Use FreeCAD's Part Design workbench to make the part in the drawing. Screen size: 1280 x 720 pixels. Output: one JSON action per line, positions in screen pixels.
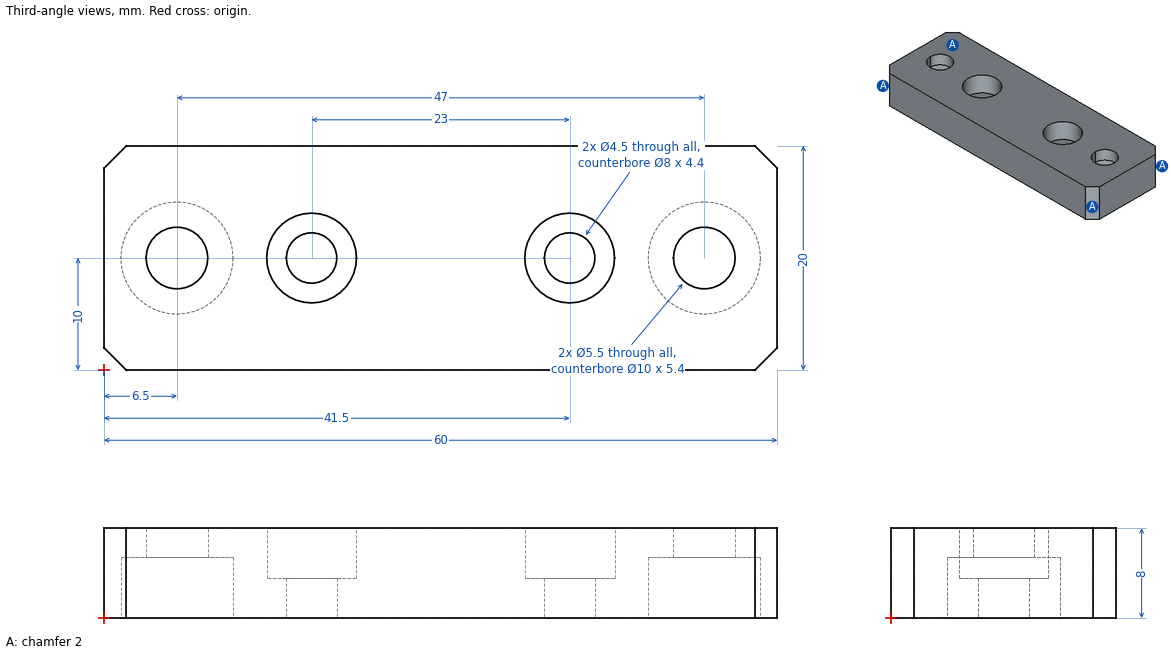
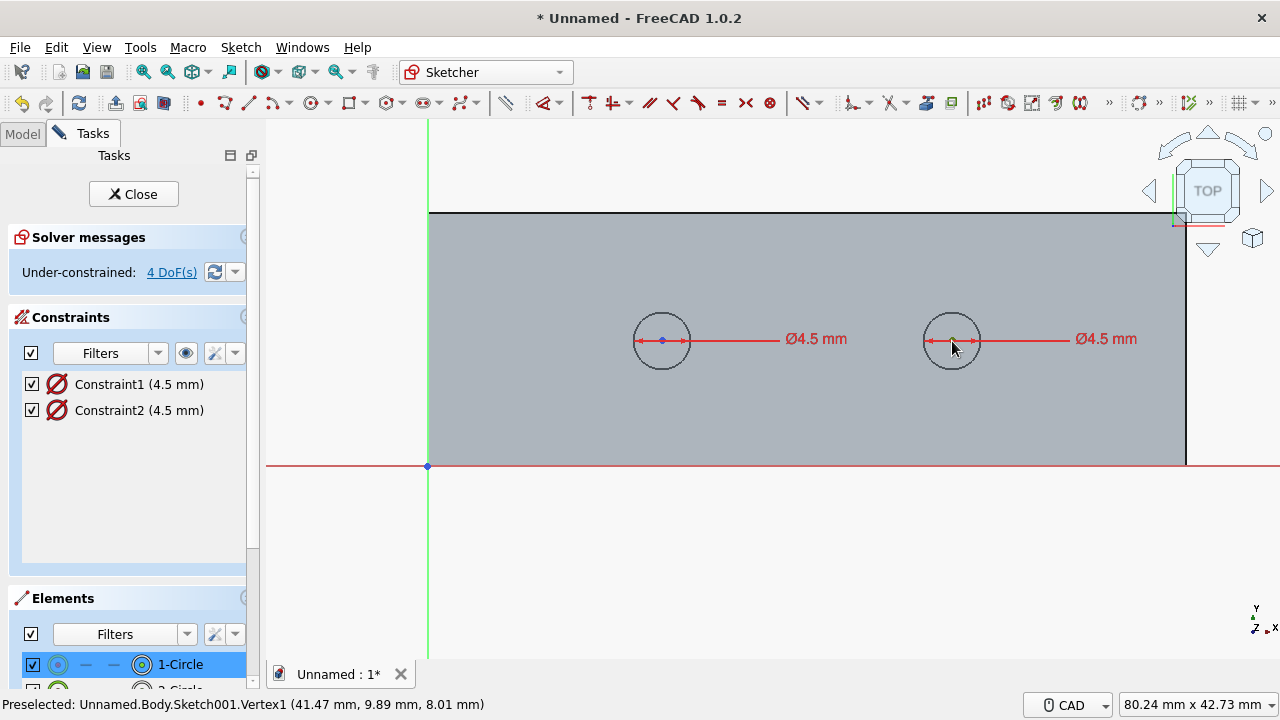
{"action": "left_click", "coordinate": [662, 341]}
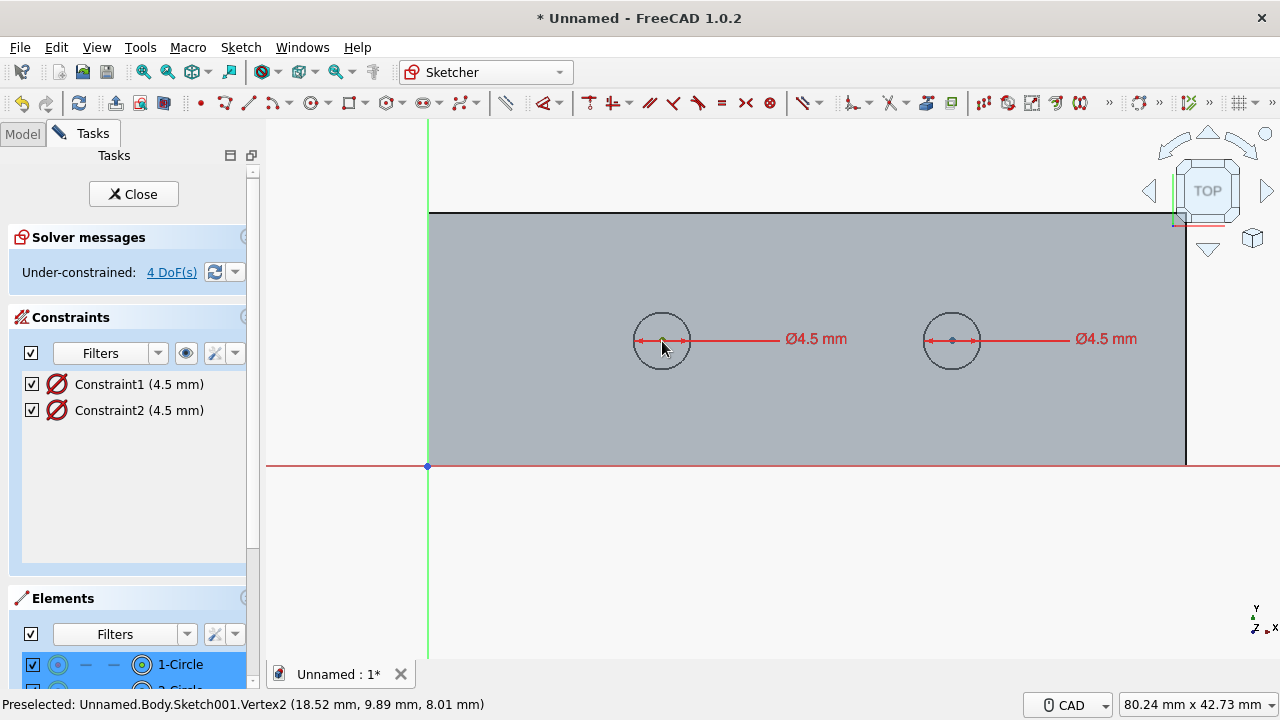
{"action": "left_click", "coordinate": [632, 104]}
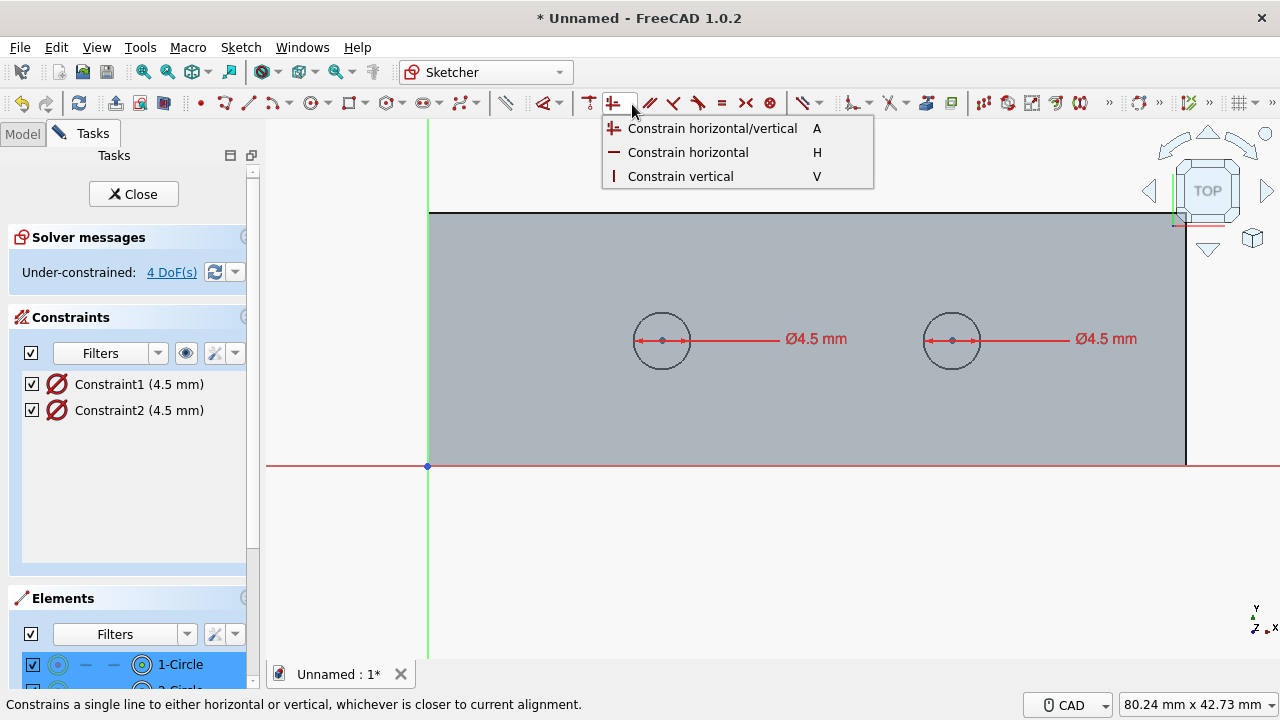
{"action": "left_click", "coordinate": [738, 152]}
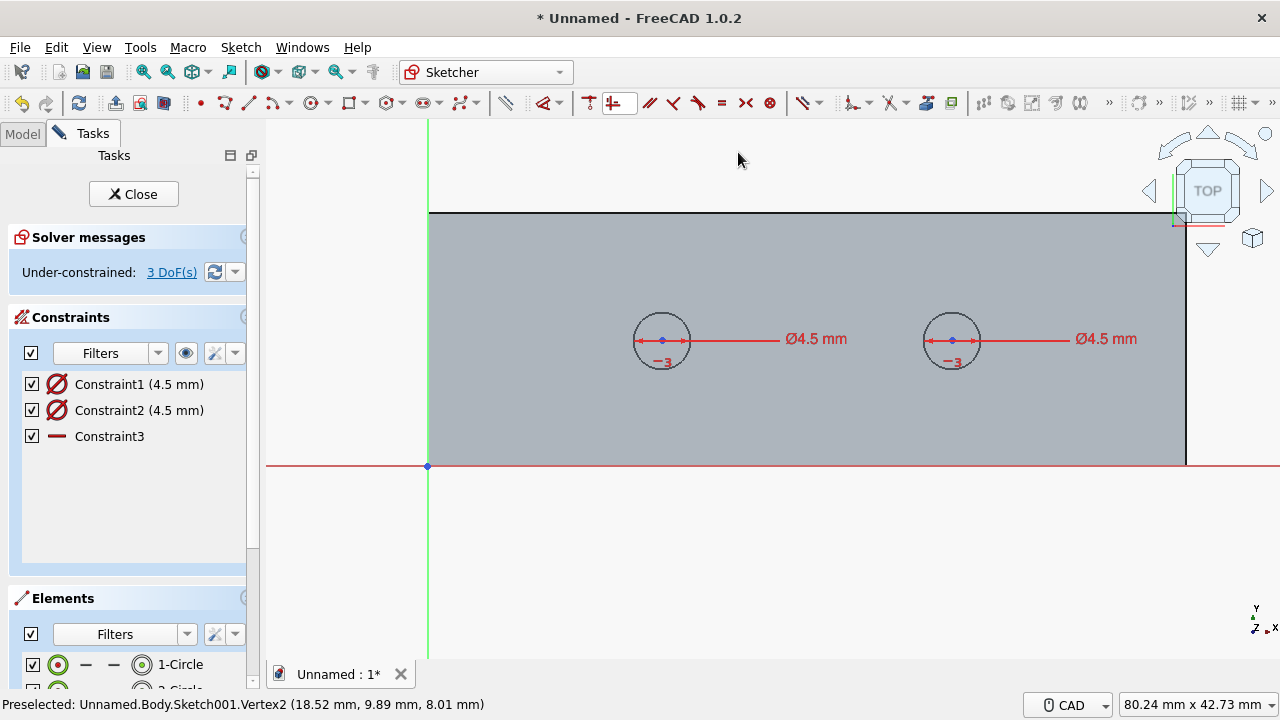
{"action": "key", "text": "d"}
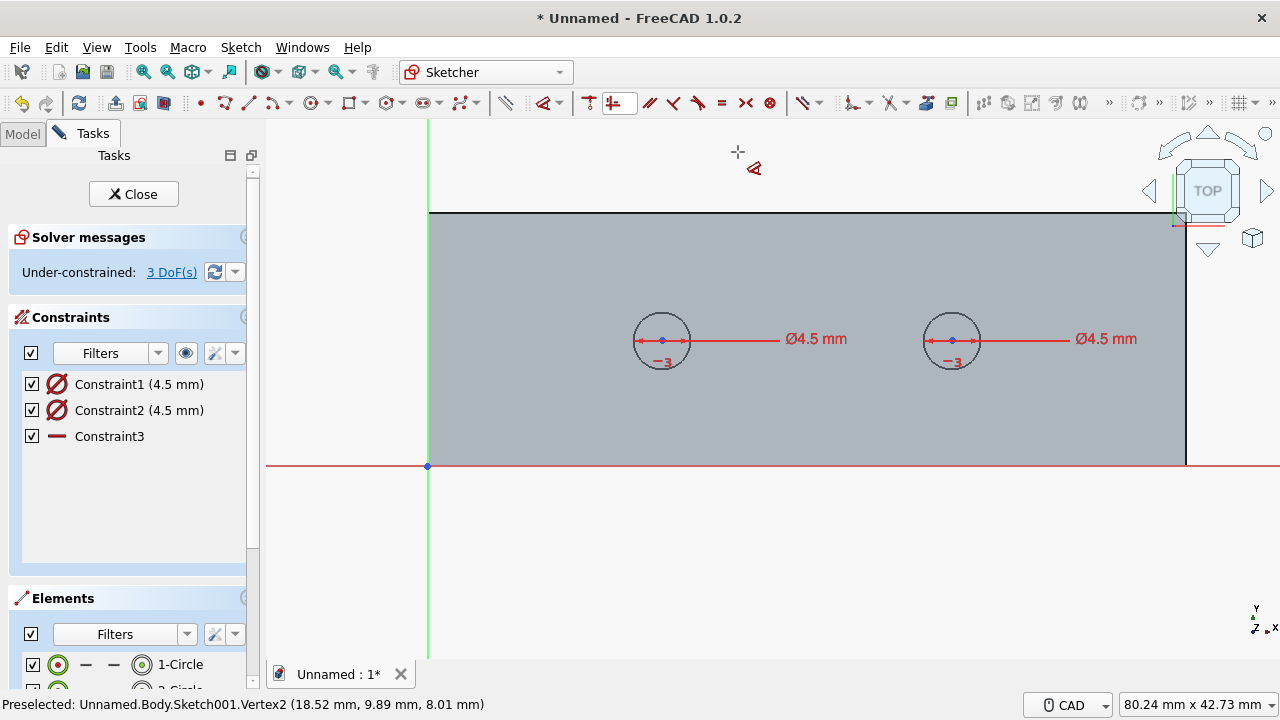
{"action": "left_click", "coordinate": [952, 341]}
{"action": "left_click", "coordinate": [394, 404]}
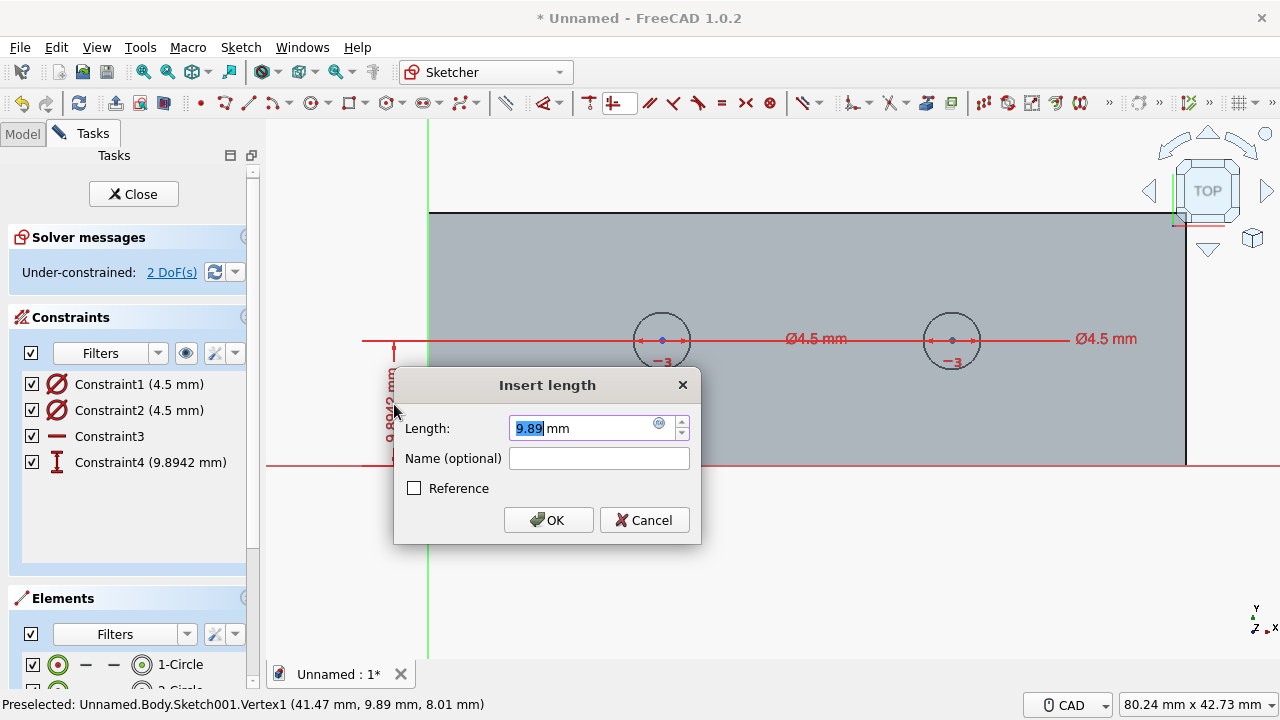
{"action": "type", "text": "10"}
{"action": "key", "text": "Return"}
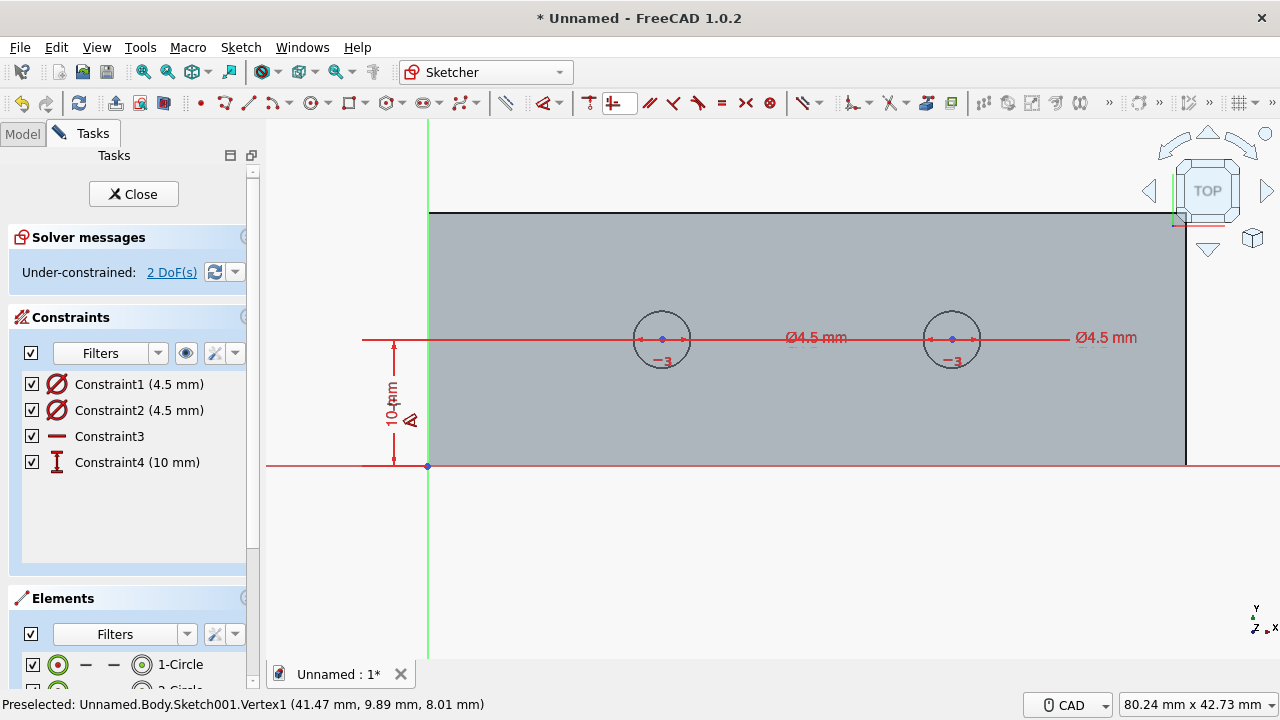
{"action": "left_click", "coordinate": [952, 340]}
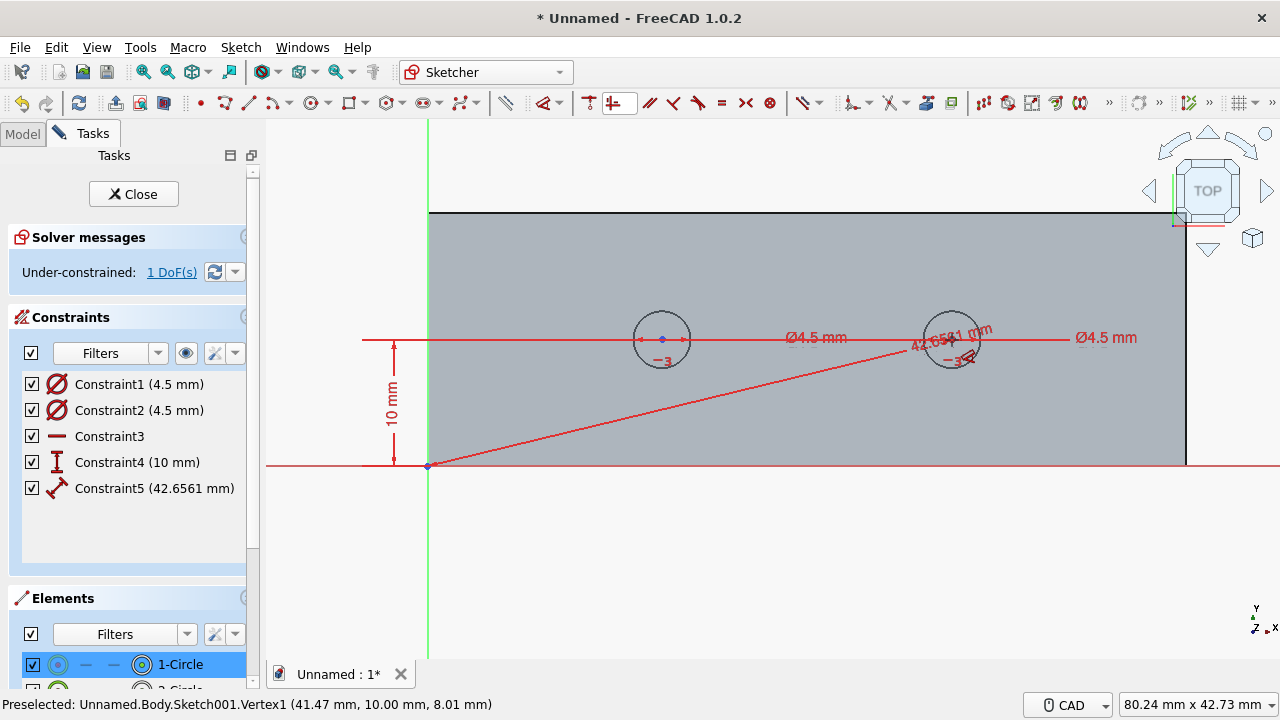
{"action": "left_click", "coordinate": [662, 340]}
{"action": "left_click", "coordinate": [807, 306]}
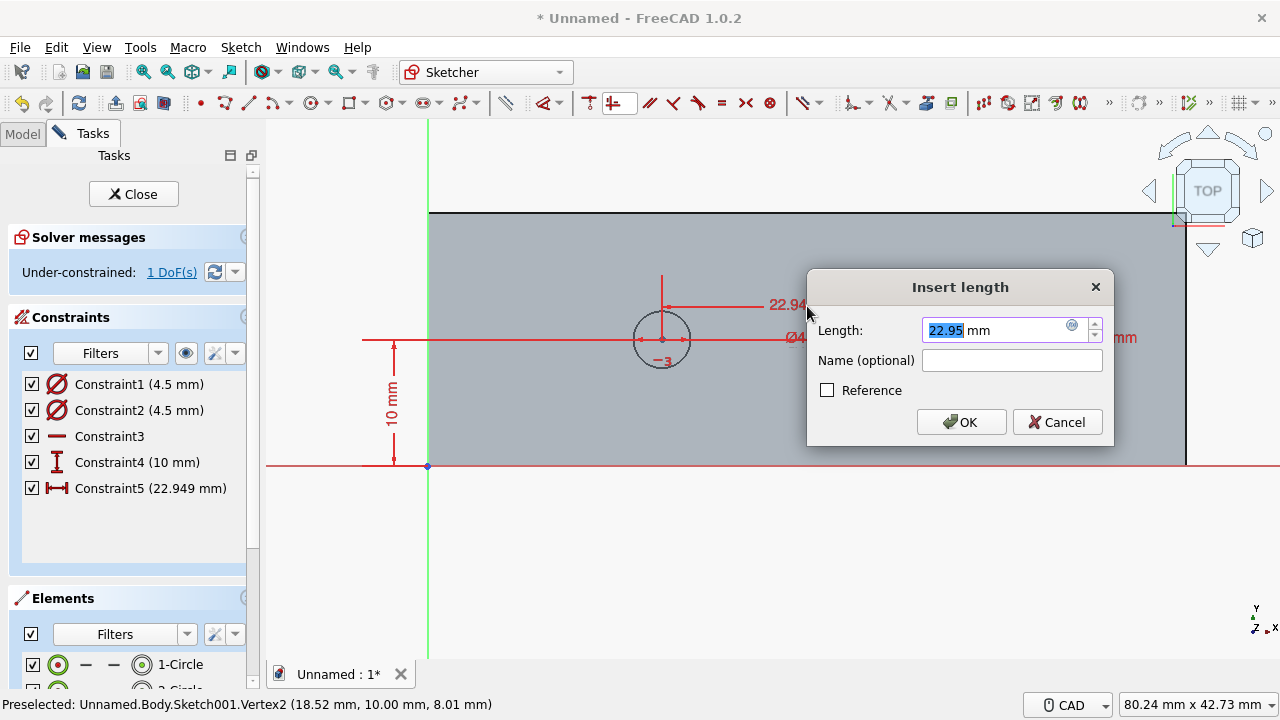
{"action": "type", "text": "23"}
{"action": "key", "text": "Return"}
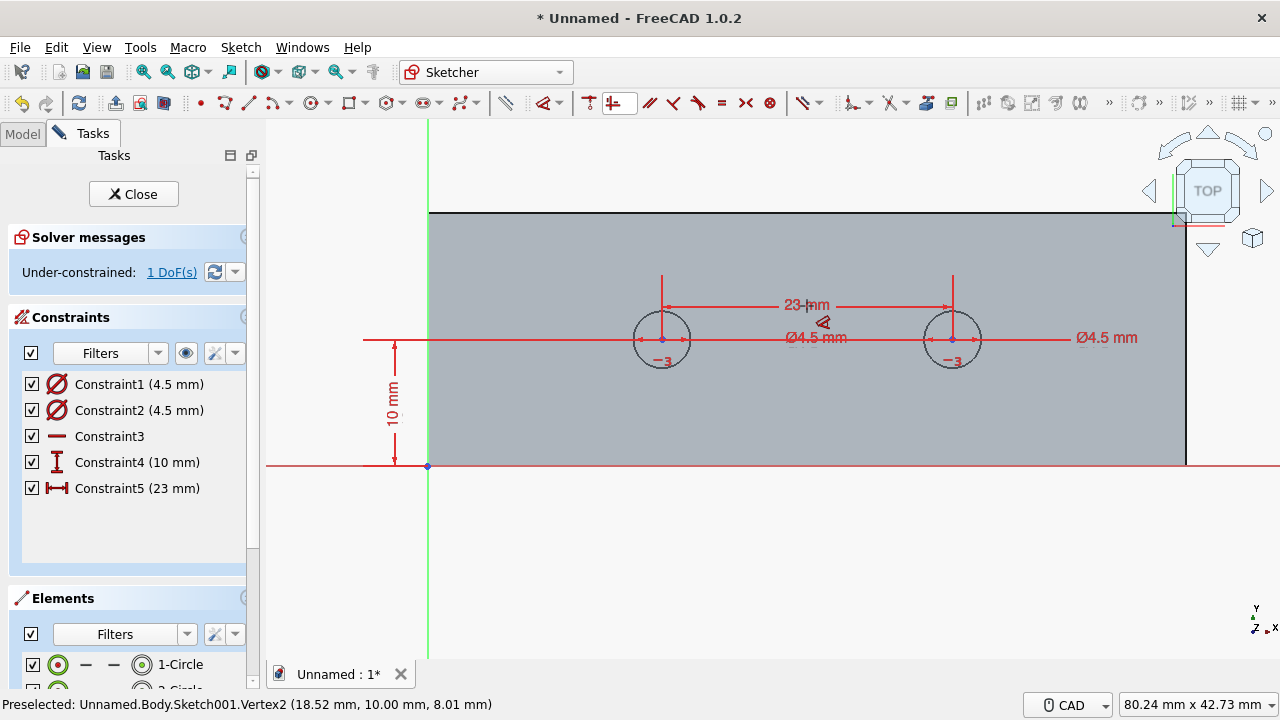
{"action": "left_click", "coordinate": [953, 340]}
{"action": "left_click", "coordinate": [690, 500]}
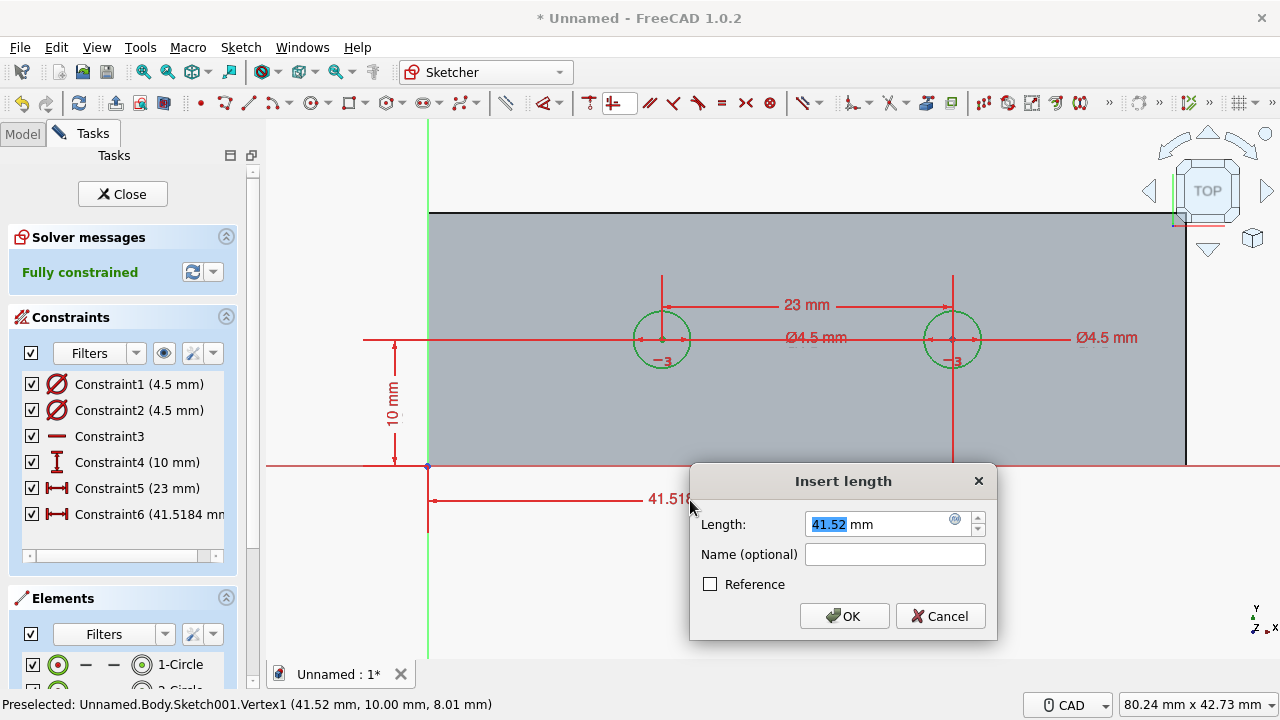
{"action": "type", "text": "41.5"}
{"action": "key", "text": "Return"}
{"action": "key", "text": "Escape"}